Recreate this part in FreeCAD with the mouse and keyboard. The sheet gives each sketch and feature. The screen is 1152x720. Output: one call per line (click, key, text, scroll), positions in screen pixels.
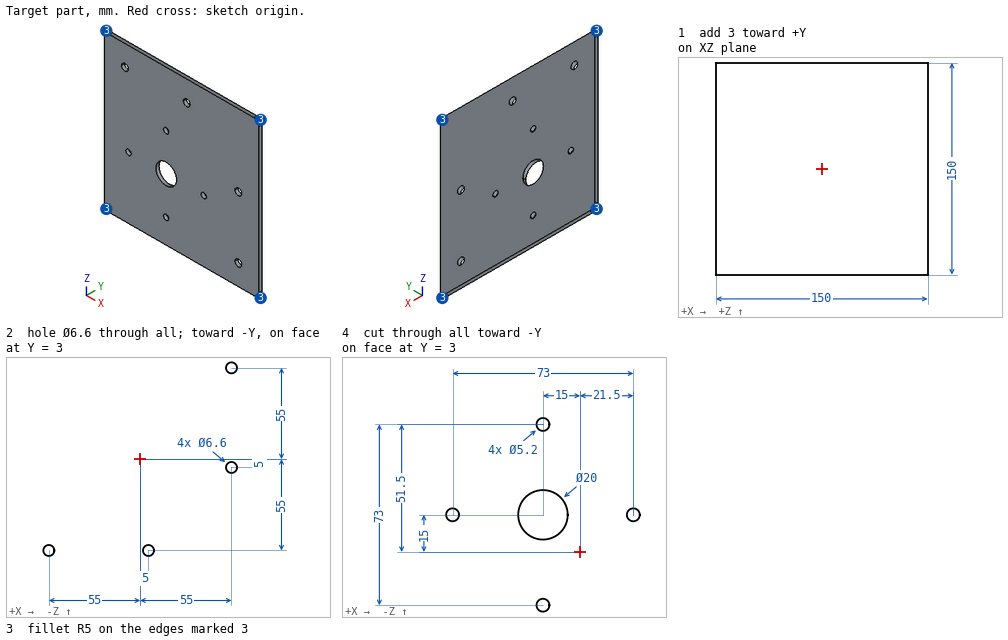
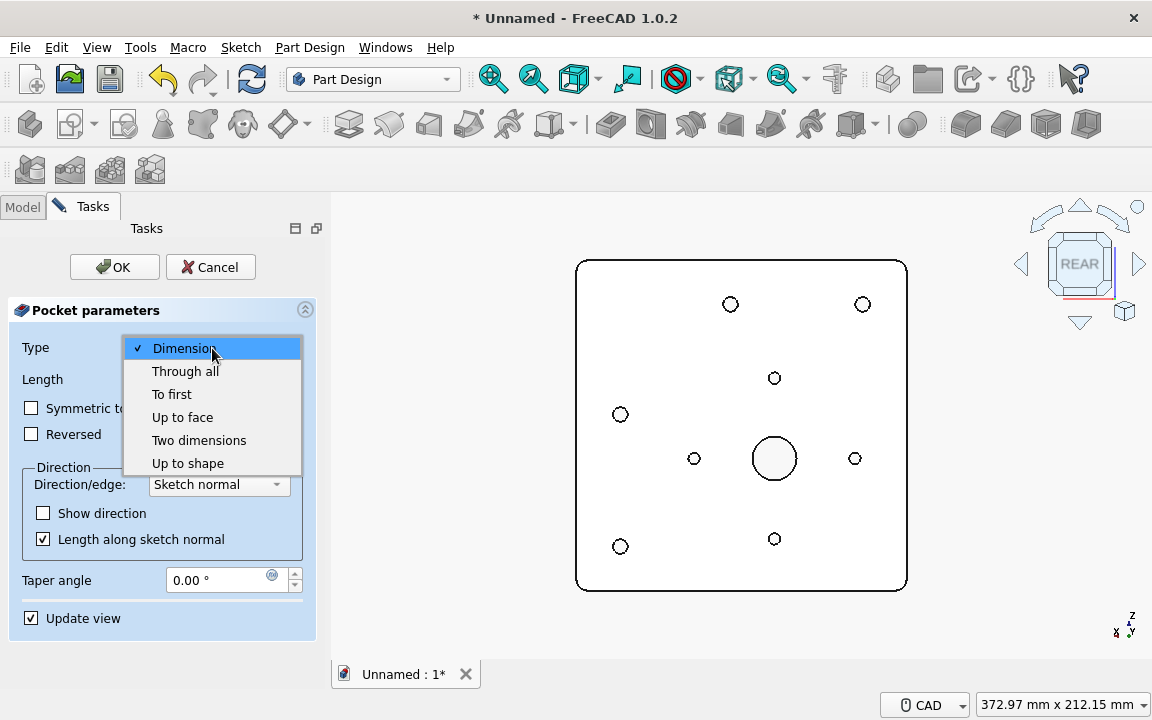
click(212, 372)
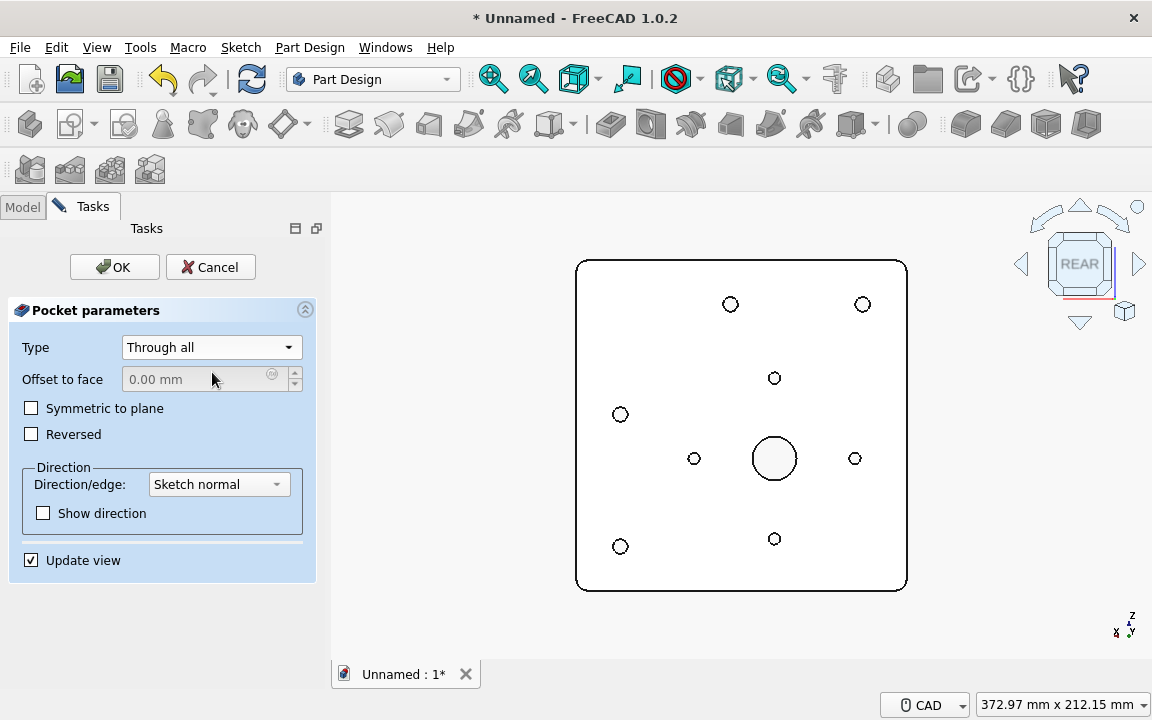
click(115, 267)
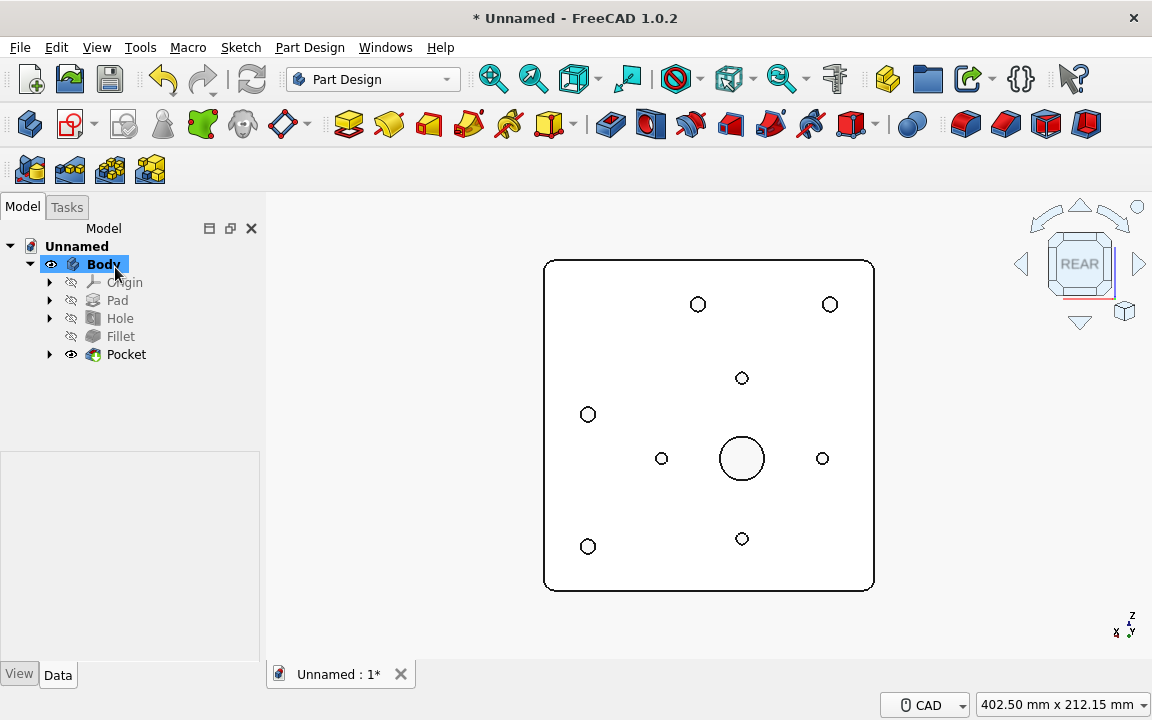
key(0)